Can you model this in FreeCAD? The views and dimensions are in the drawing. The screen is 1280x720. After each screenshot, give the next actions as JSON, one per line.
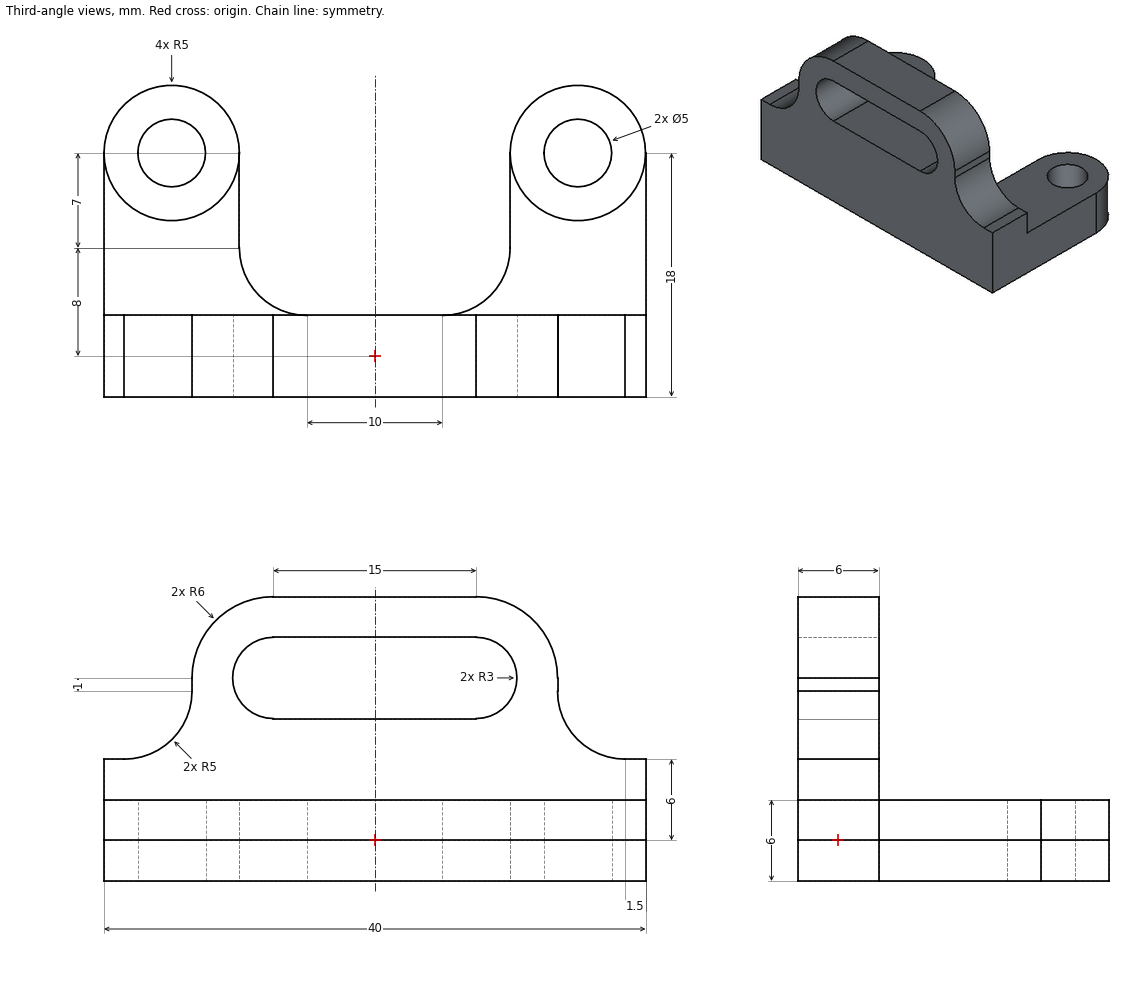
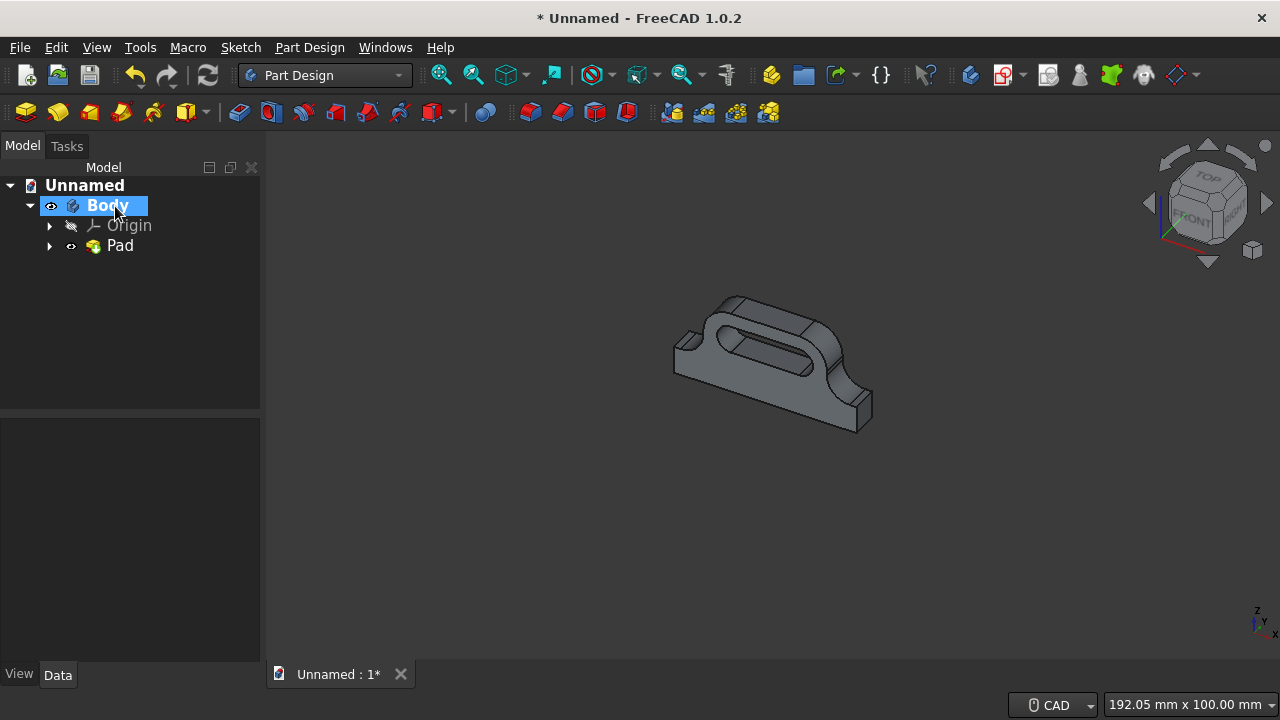
{"action": "left_click", "coordinate": [442, 76]}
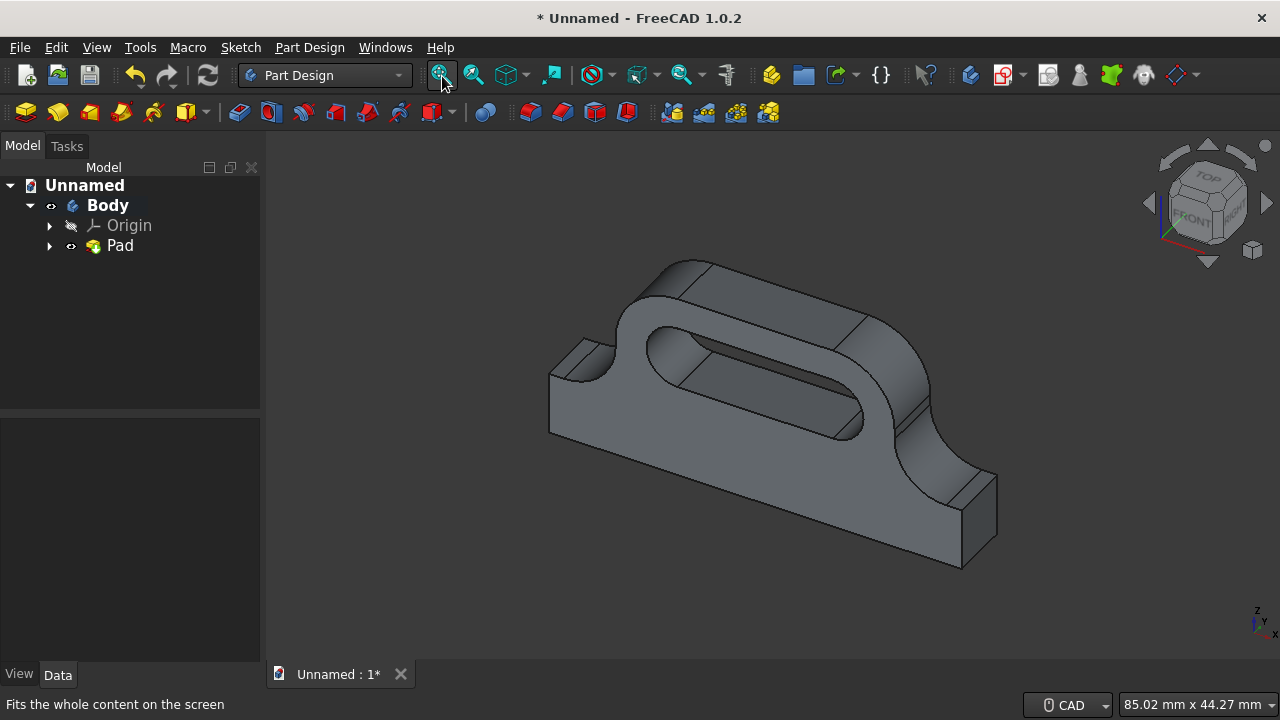
{"action": "key", "text": "5"}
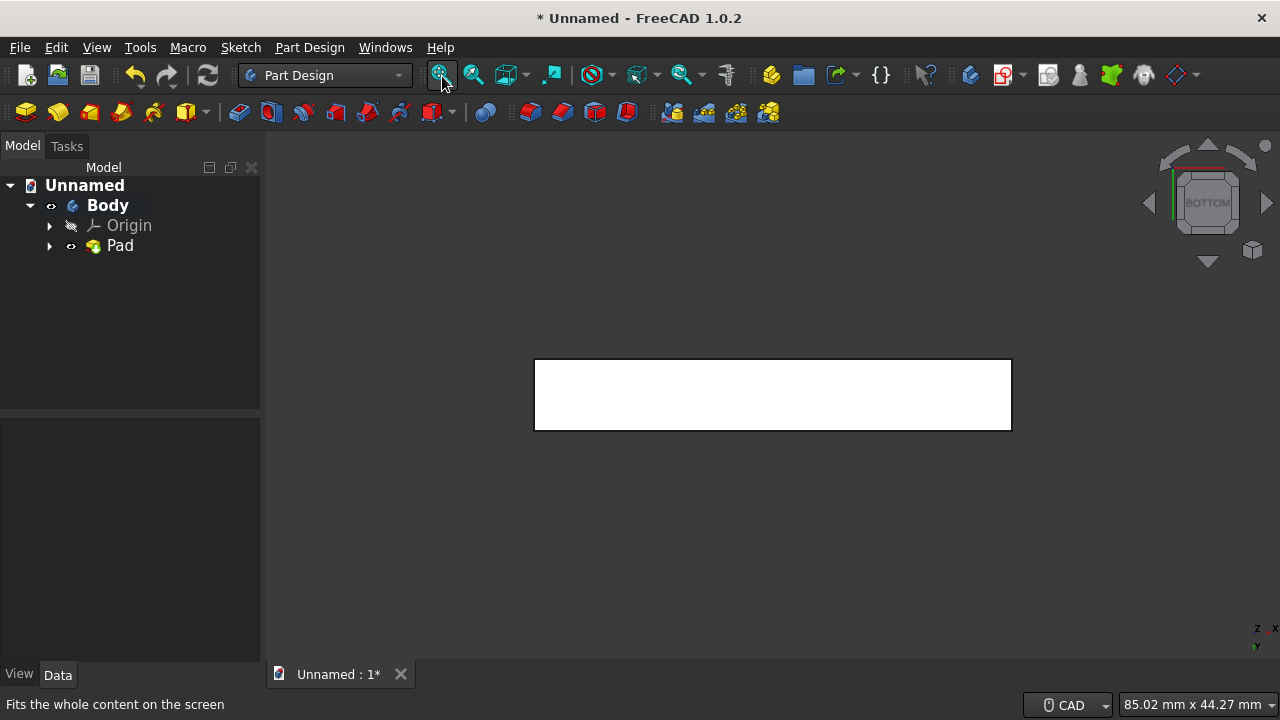
{"action": "left_click", "coordinate": [909, 394]}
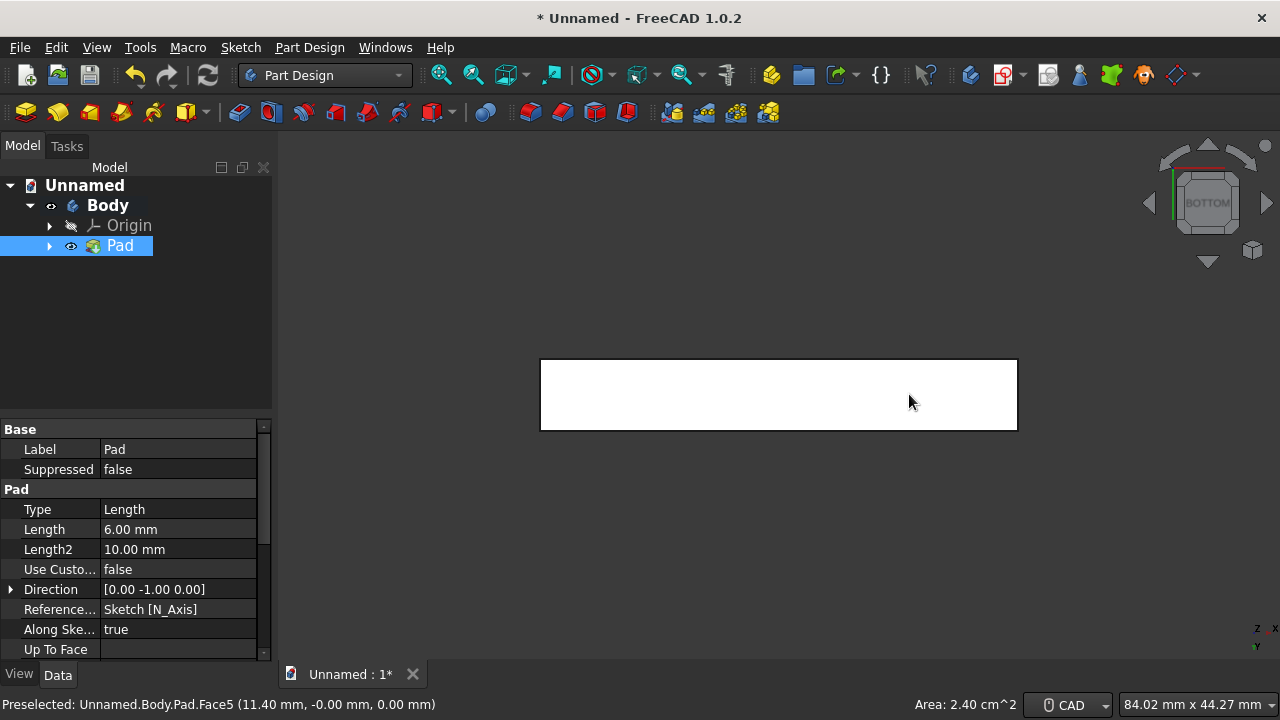
{"action": "left_click", "coordinate": [1004, 76]}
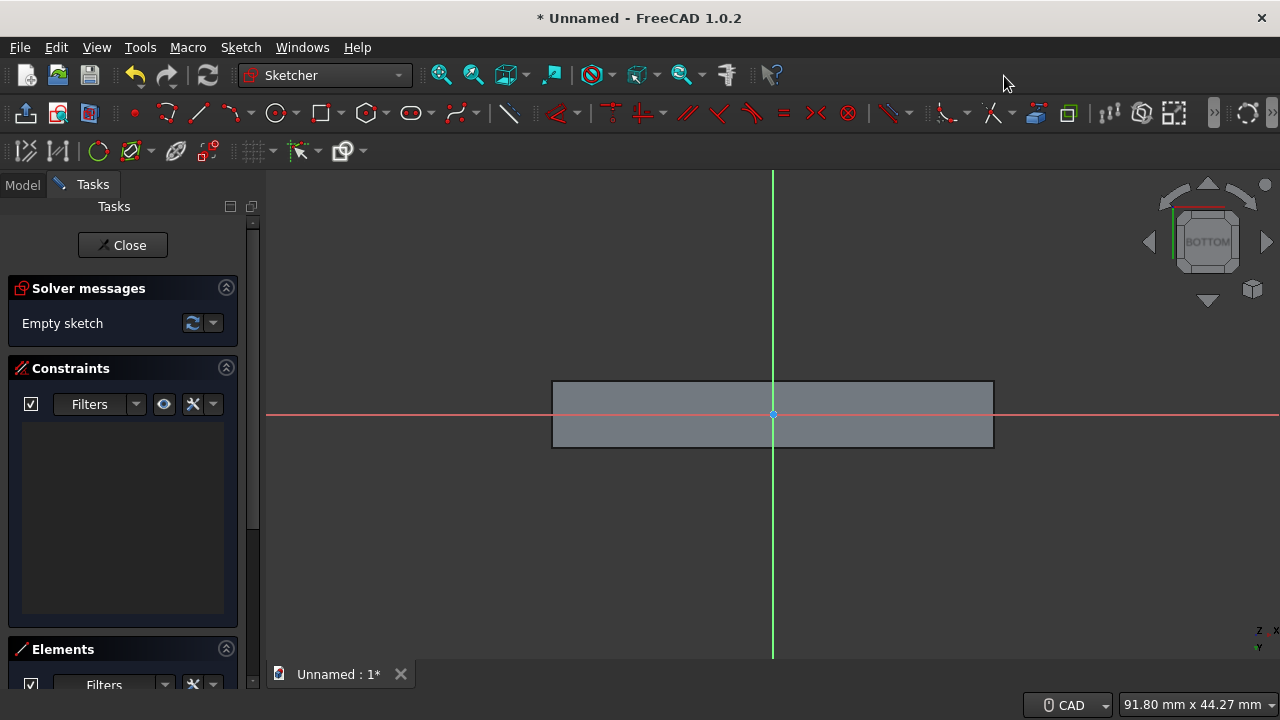
{"action": "scroll", "coordinate": [395, 198], "scroll_direction": "down", "scroll_amount": 1}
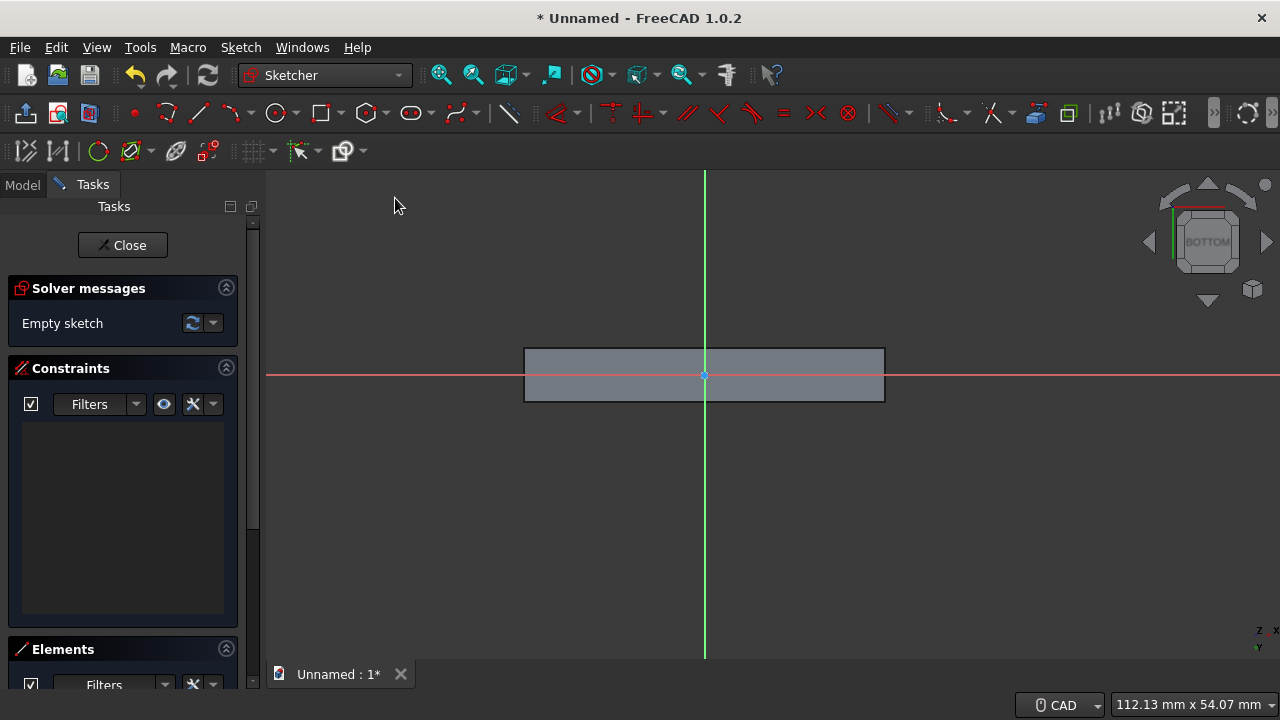
{"action": "scroll", "coordinate": [705, 529], "scroll_direction": "up", "scroll_amount": 2}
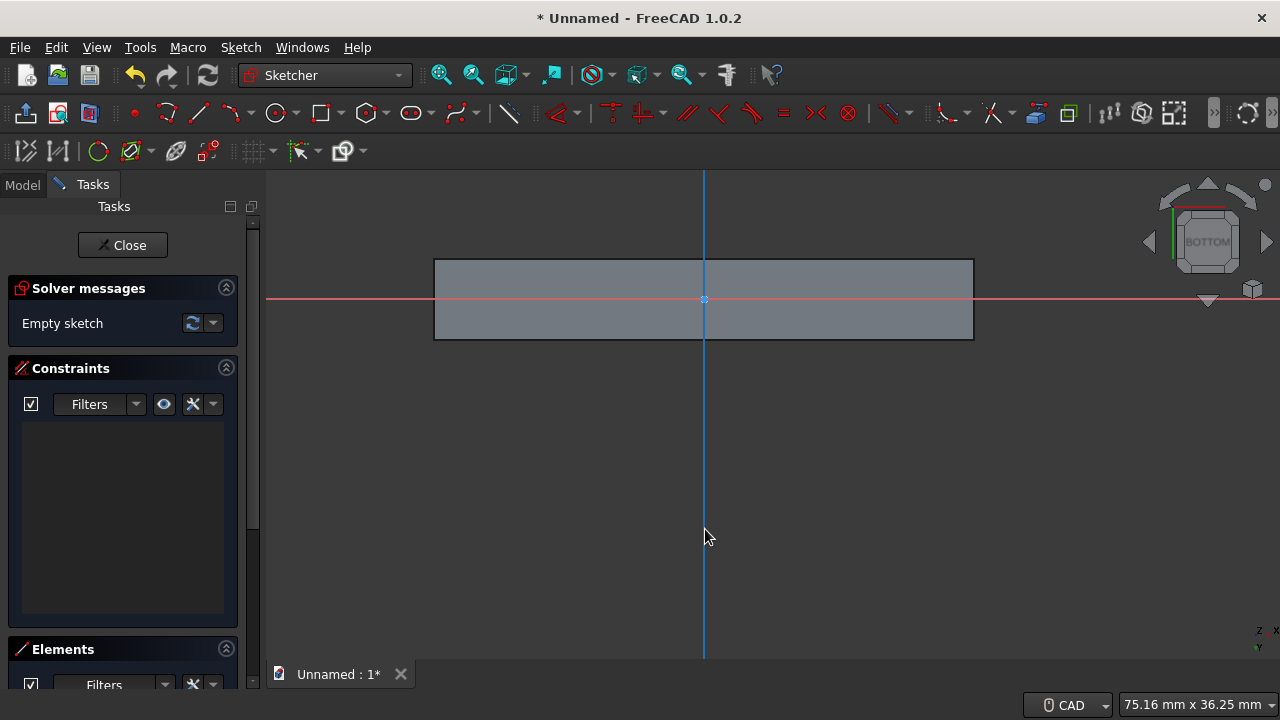
{"action": "left_click", "coordinate": [200, 114]}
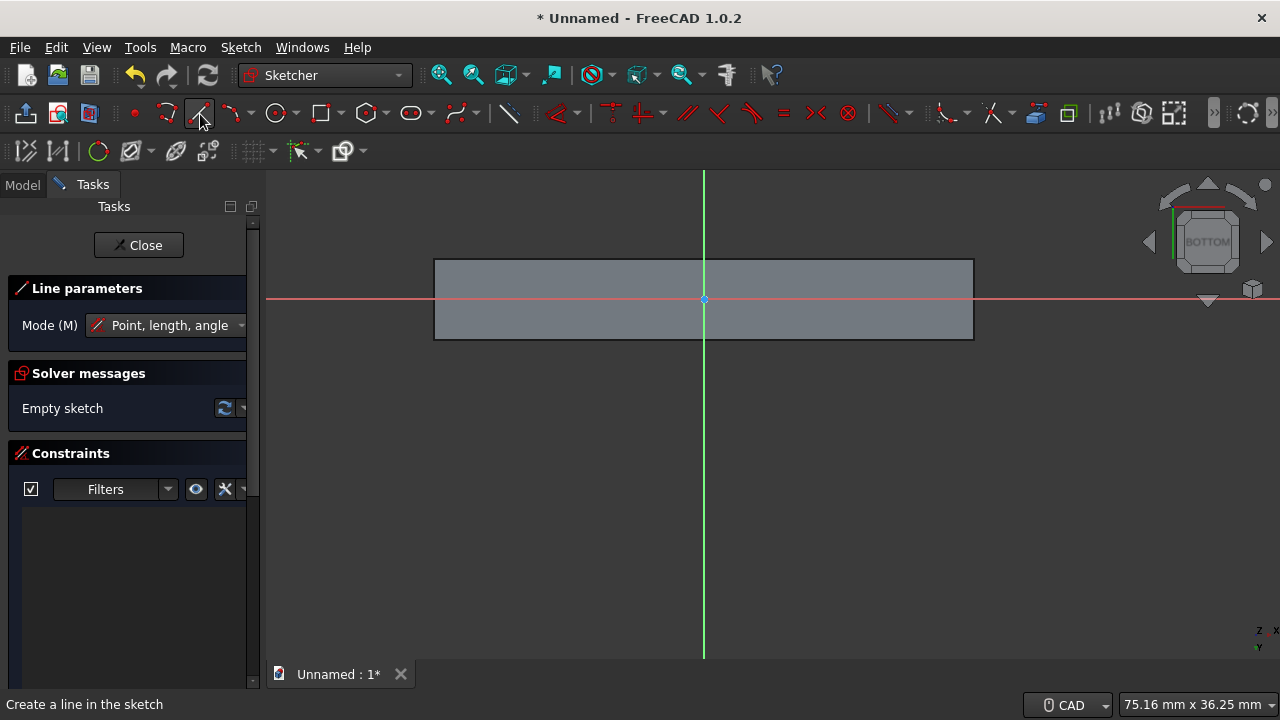
{"action": "left_click", "coordinate": [569, 502]}
{"action": "left_click", "coordinate": [569, 407]}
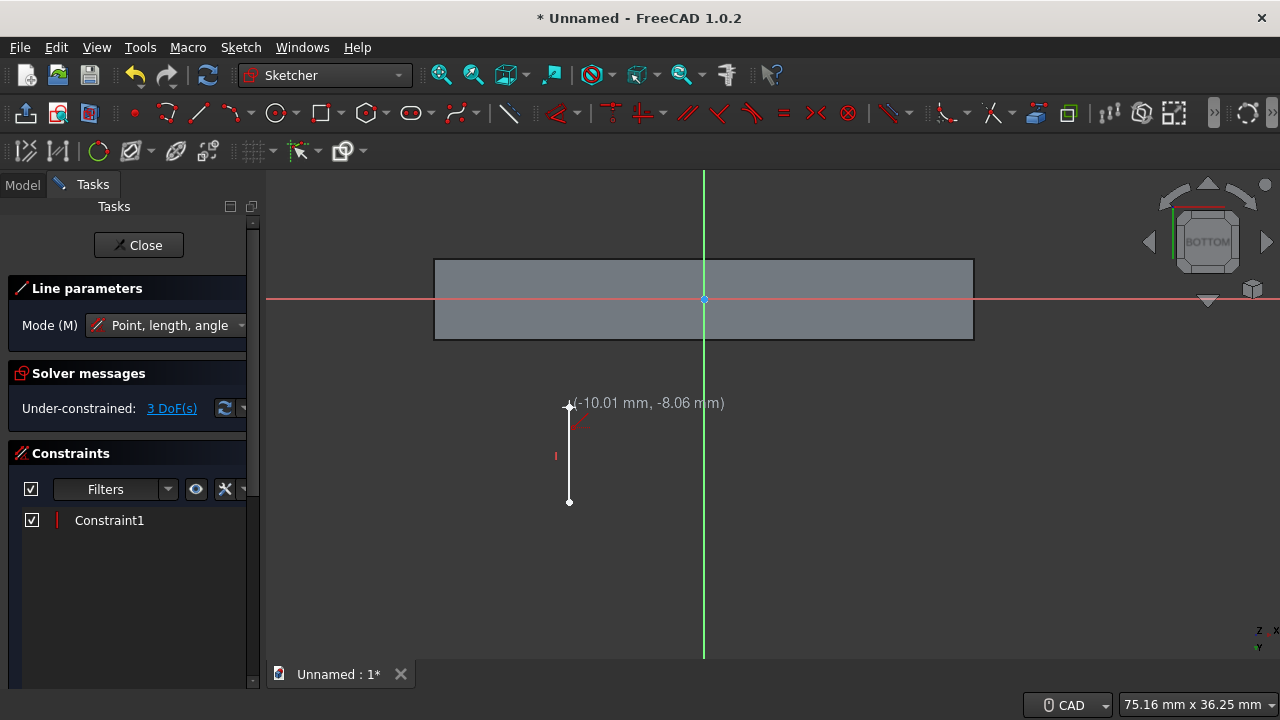
{"action": "left_click", "coordinate": [637, 340]}
{"action": "left_click", "coordinate": [772, 340]}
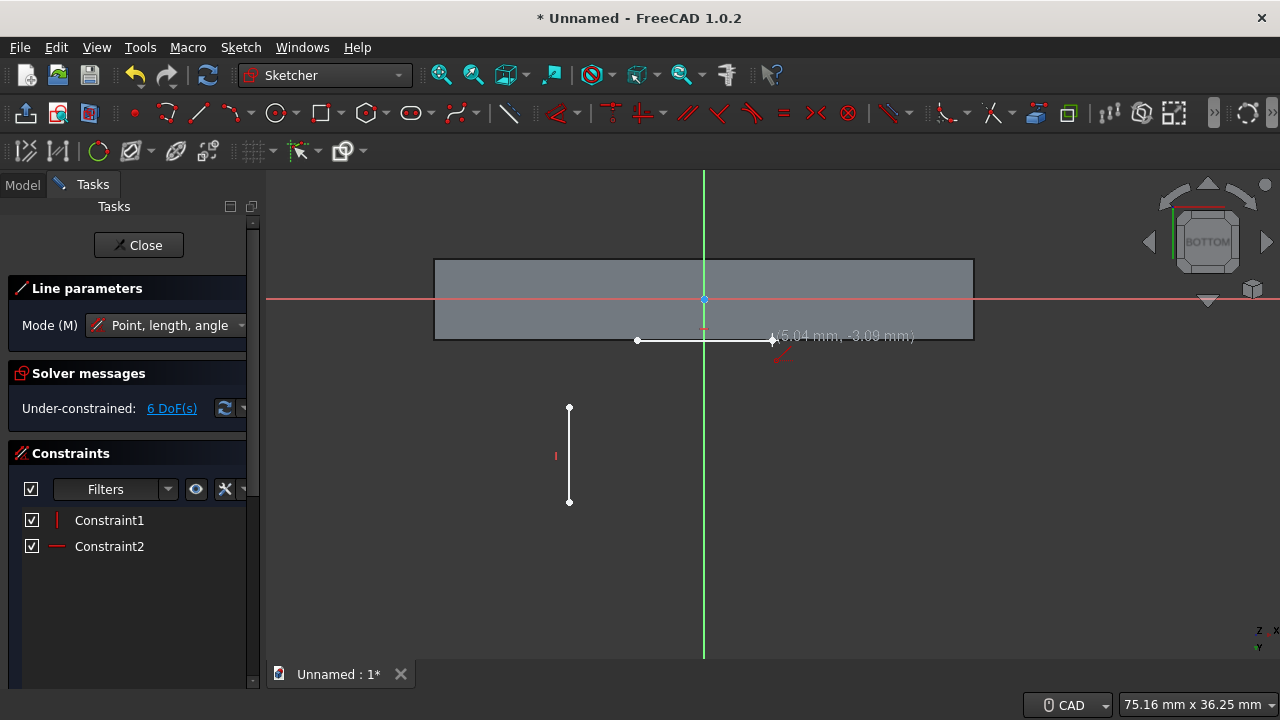
{"action": "left_click", "coordinate": [839, 407]}
{"action": "left_click", "coordinate": [839, 502]}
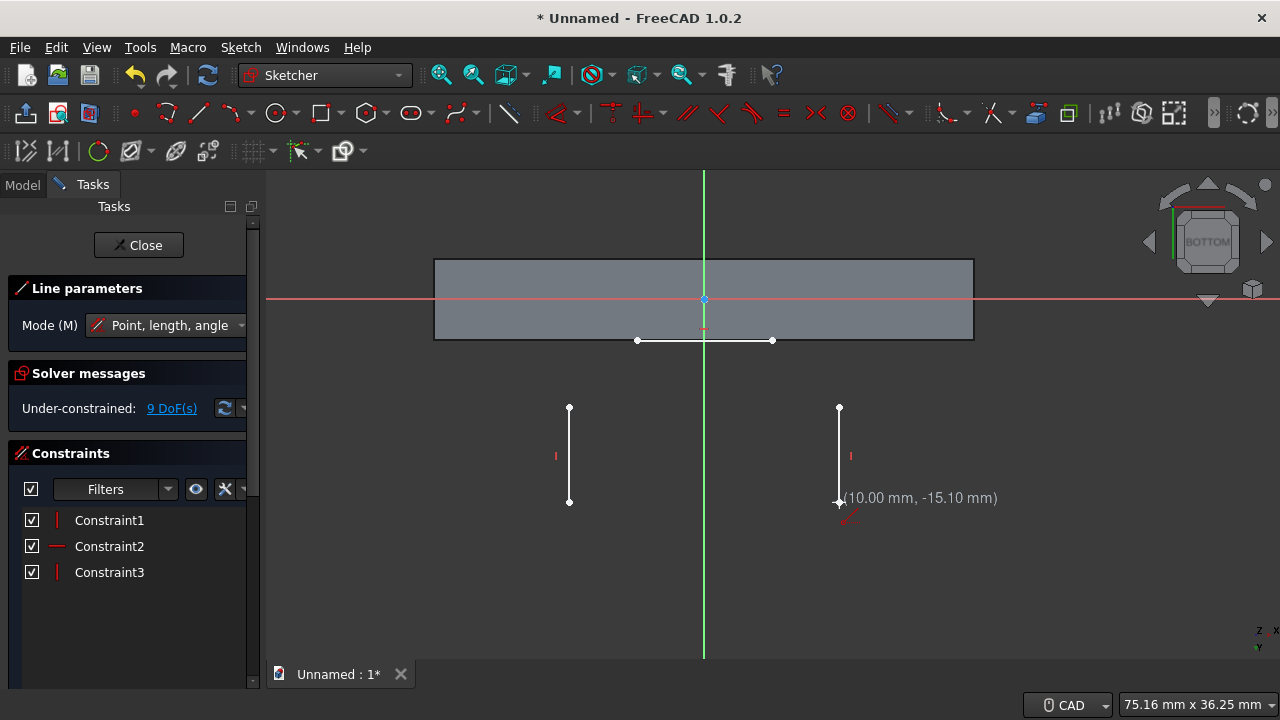
{"action": "left_click", "coordinate": [168, 114]}